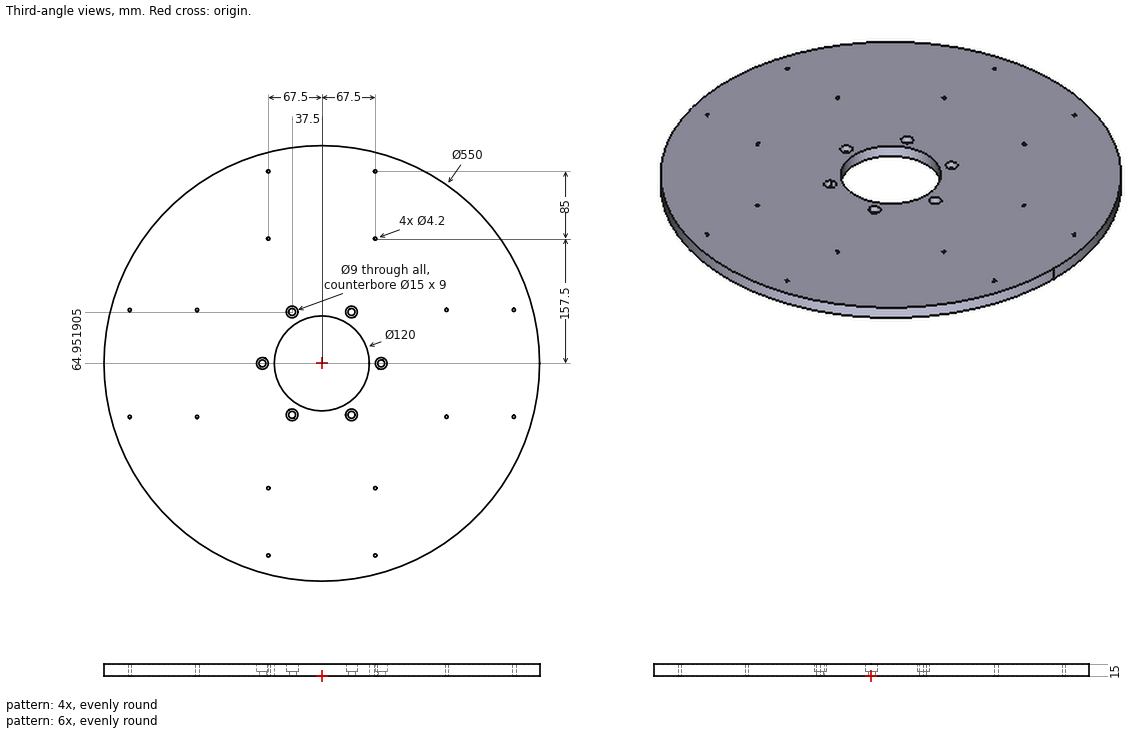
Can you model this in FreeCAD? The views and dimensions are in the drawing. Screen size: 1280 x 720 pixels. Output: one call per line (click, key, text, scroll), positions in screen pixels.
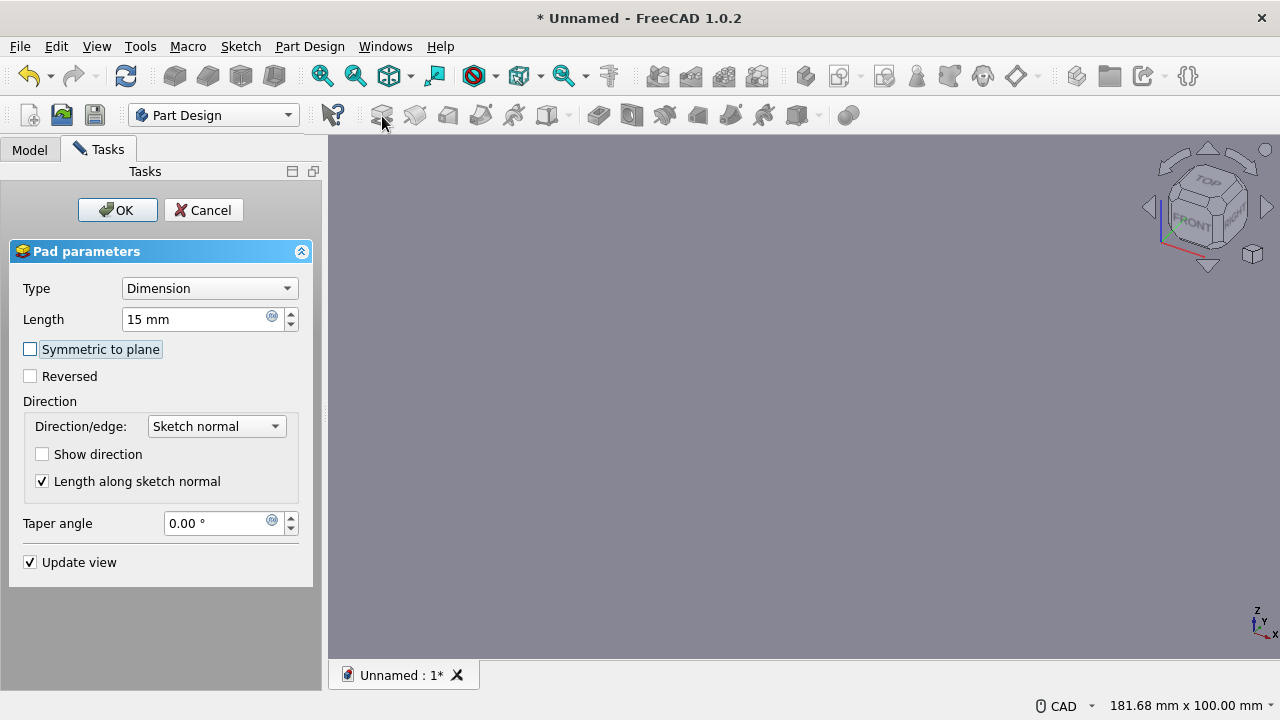
click(118, 210)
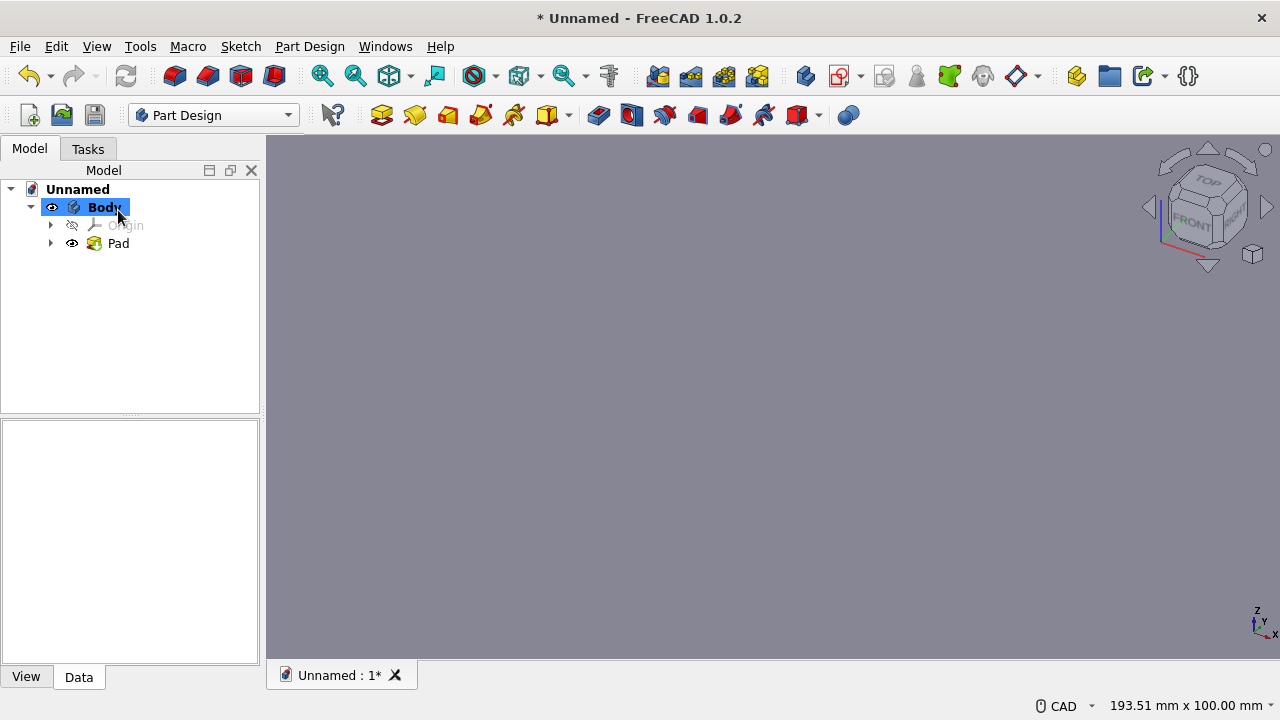
click(323, 76)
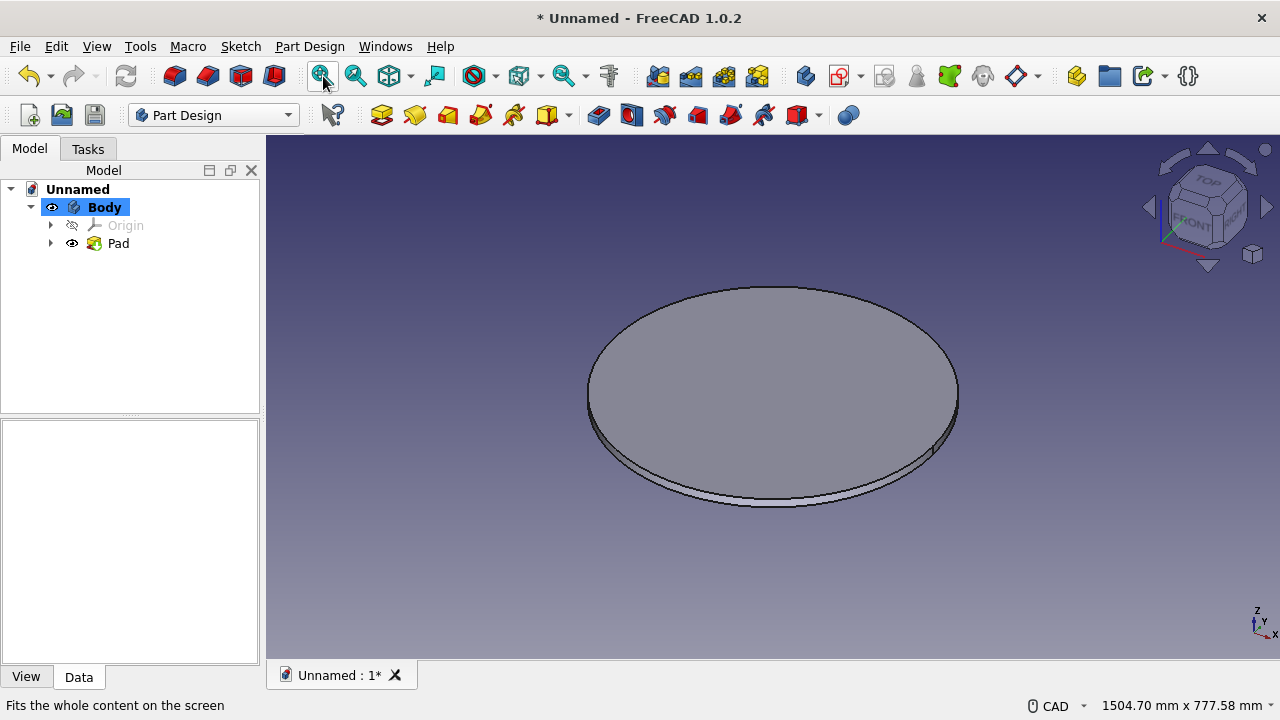
click(773, 392)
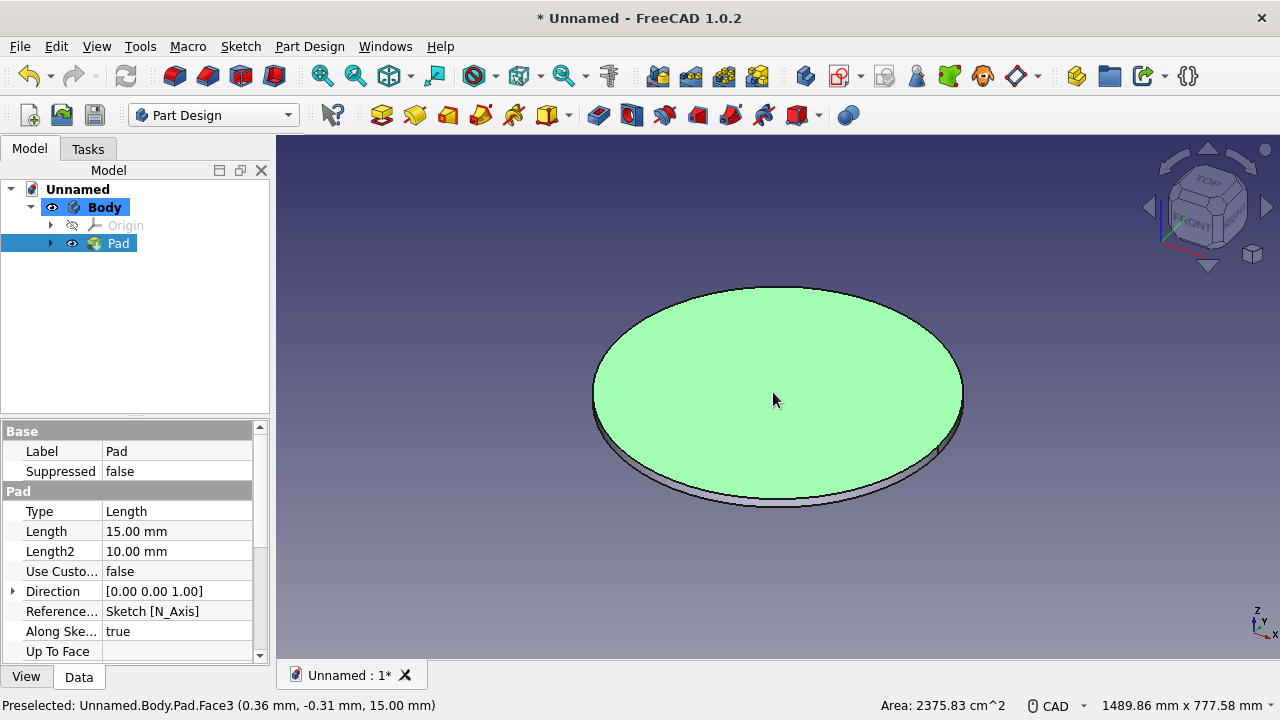
click(838, 76)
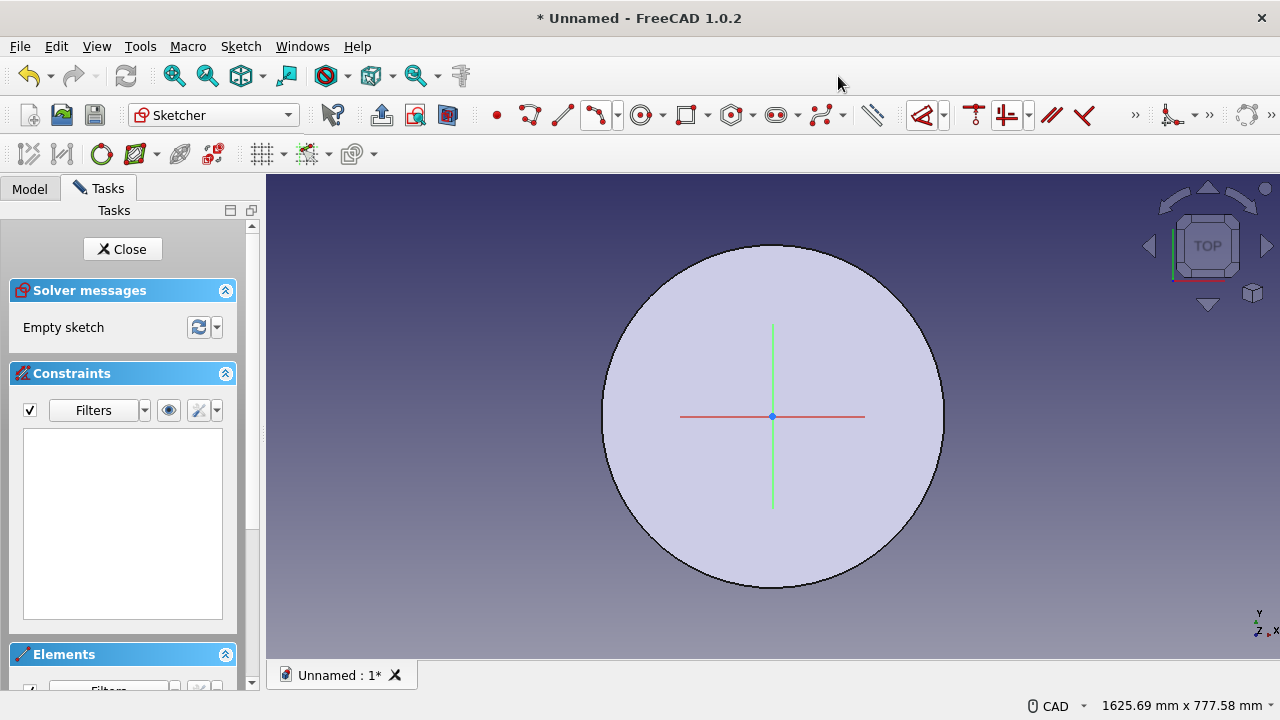
scroll(795, 416, up, 7)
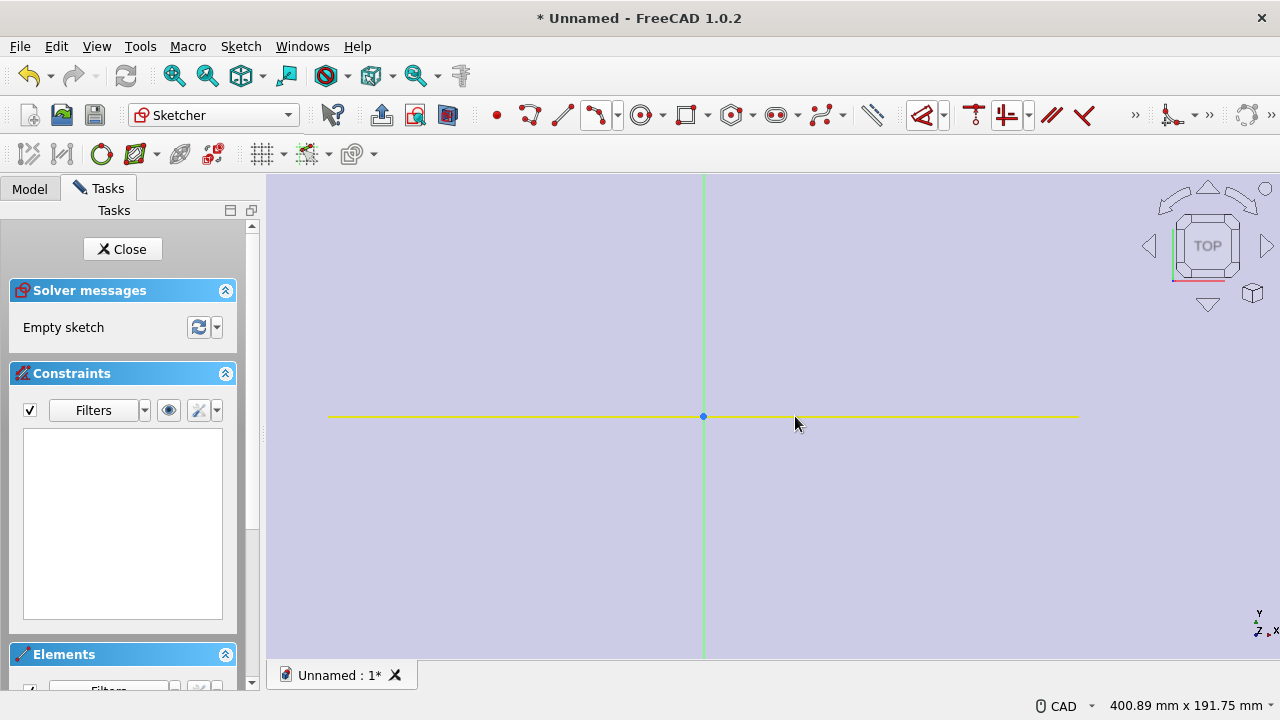
click(640, 116)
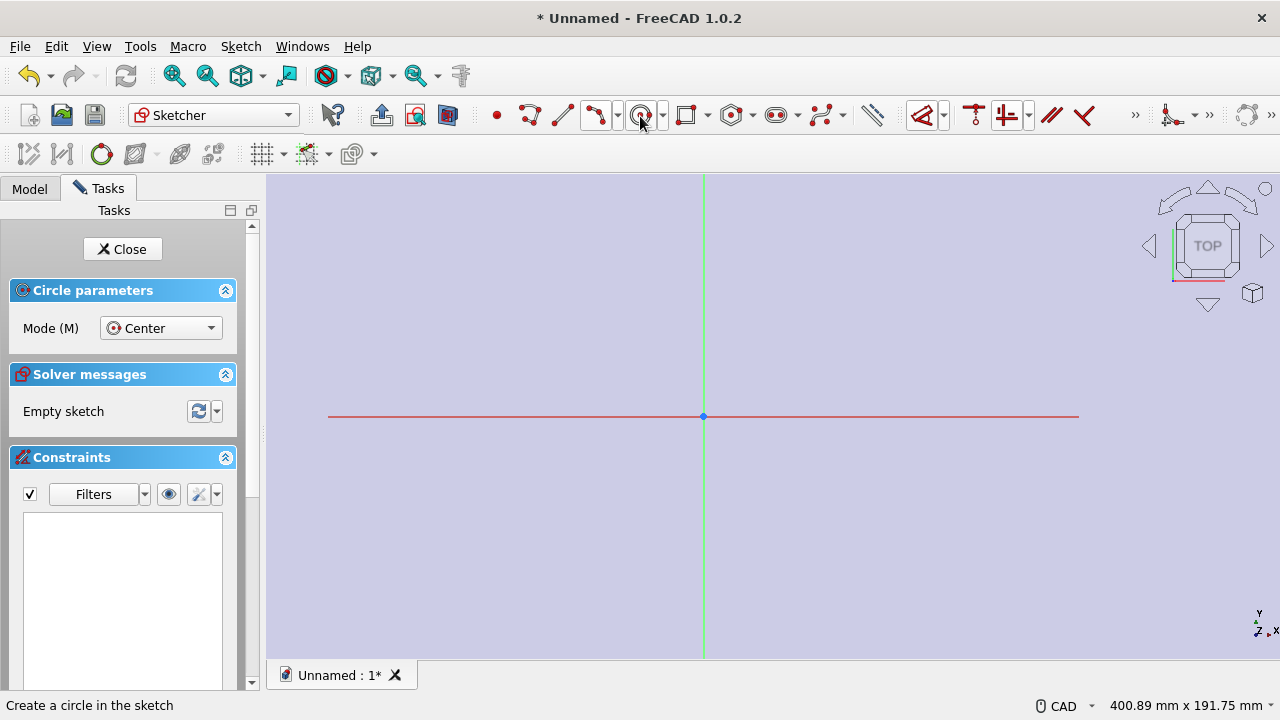
click(704, 416)
move(811, 309)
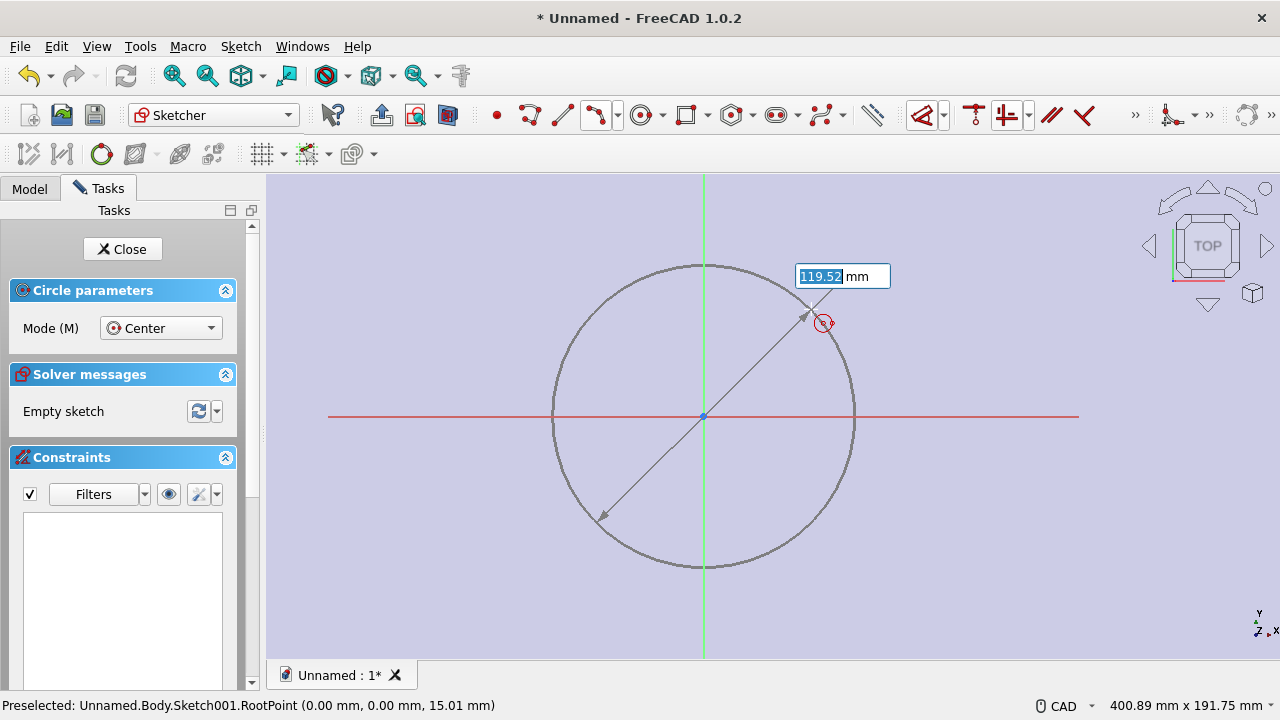
text(120)
key(Return)
key(Escape)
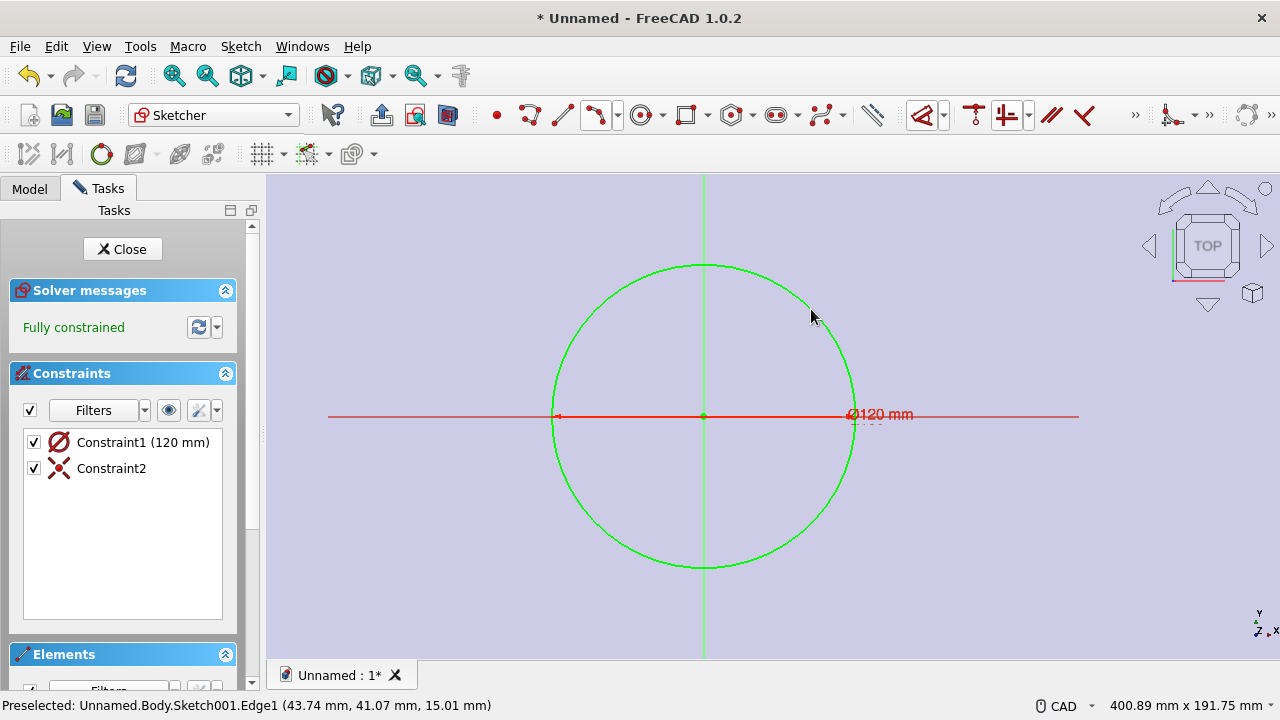
click(123, 249)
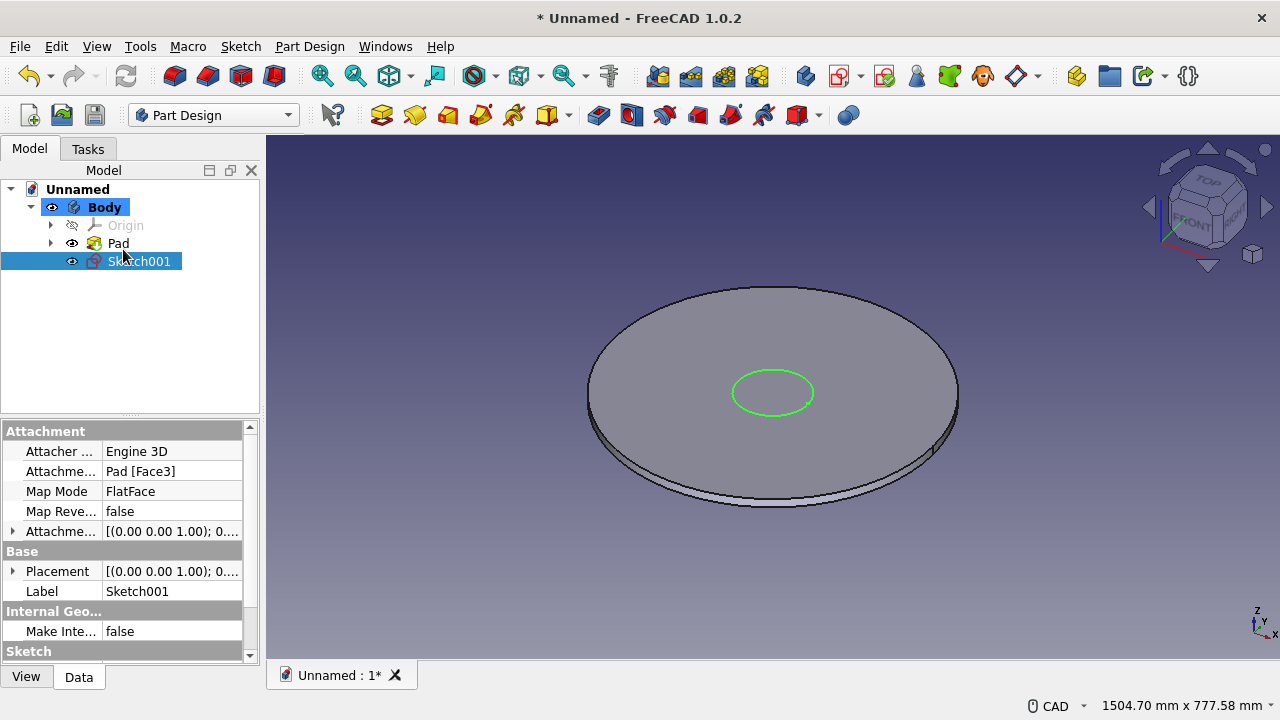
click(599, 116)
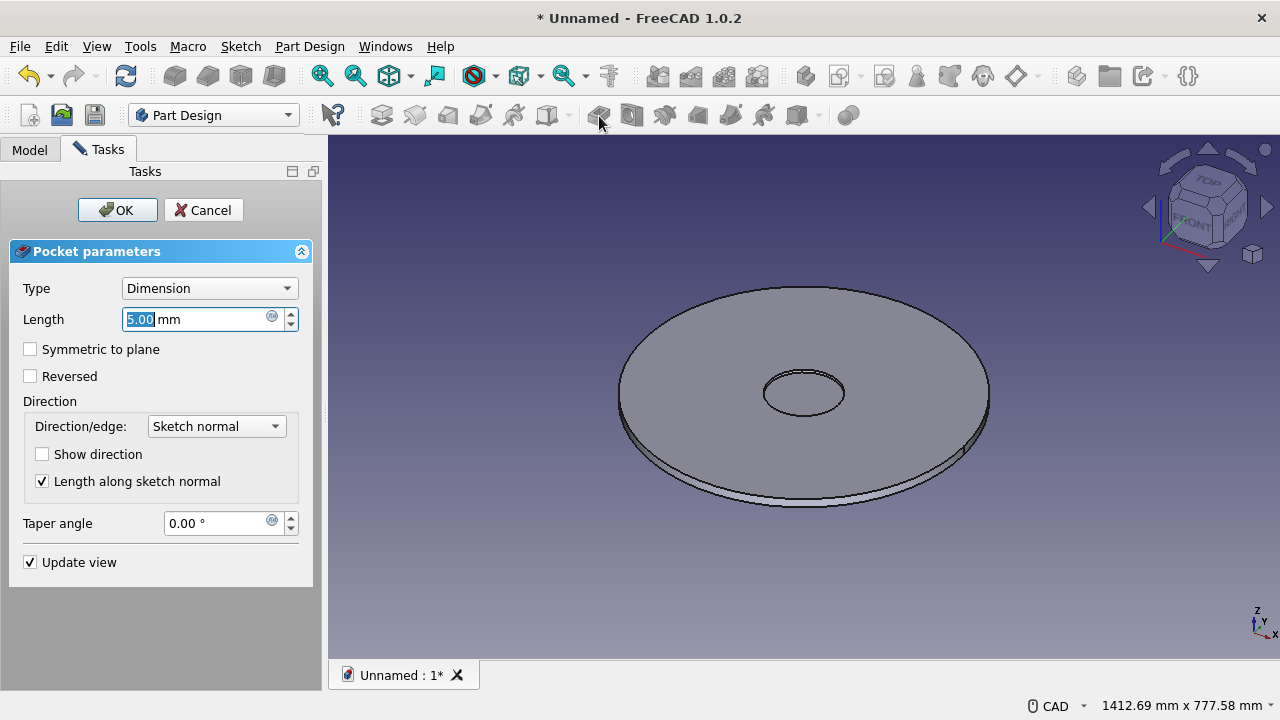
click(210, 288)